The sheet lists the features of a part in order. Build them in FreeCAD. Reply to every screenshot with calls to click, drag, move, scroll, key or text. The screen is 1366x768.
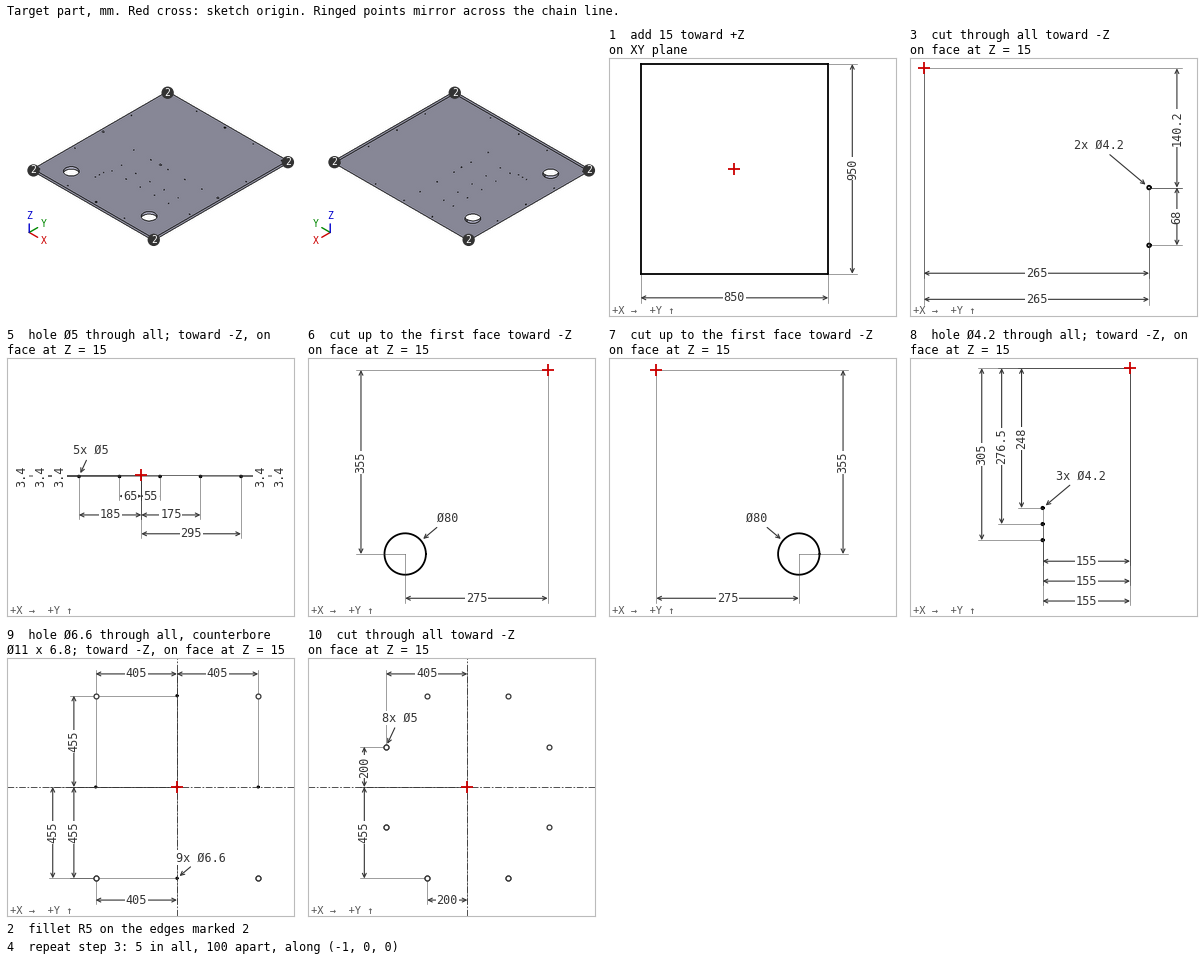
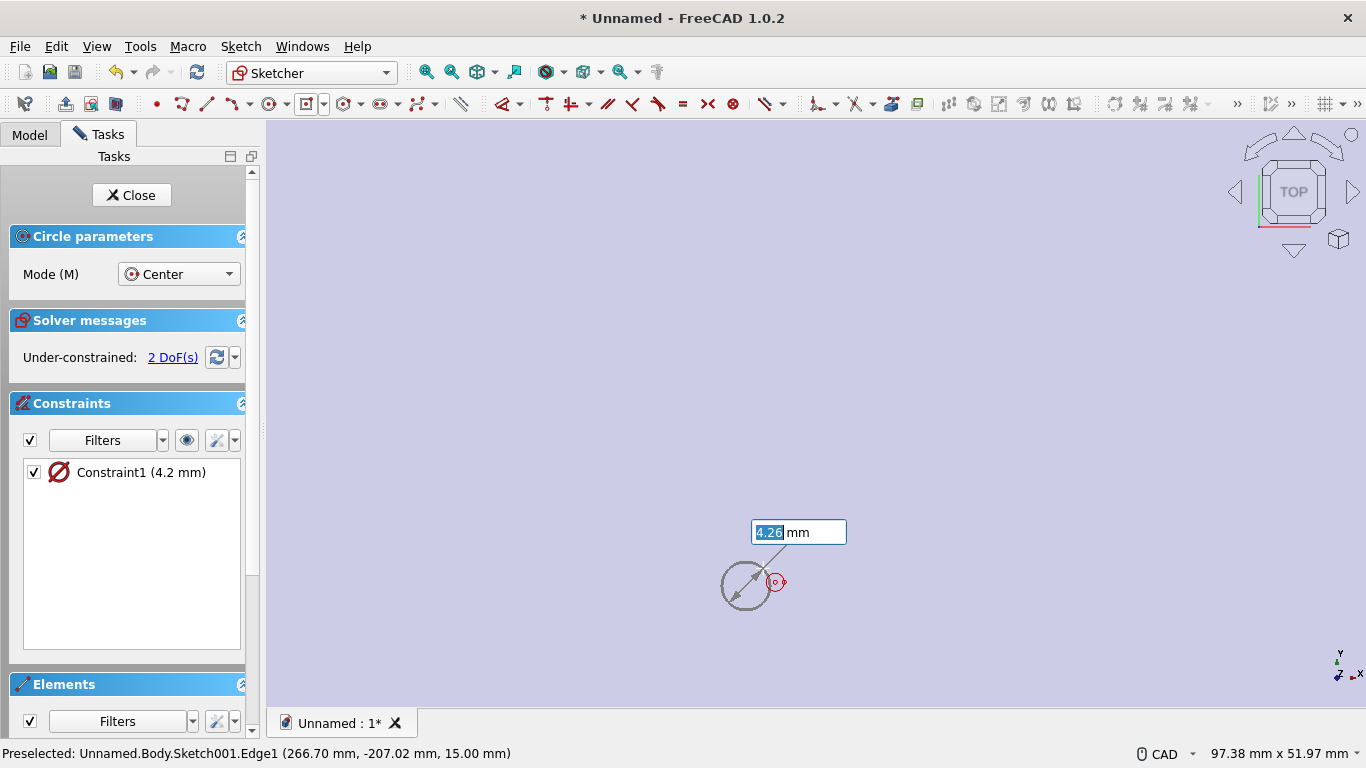
text(4.2)
key(Return)
key(Escape)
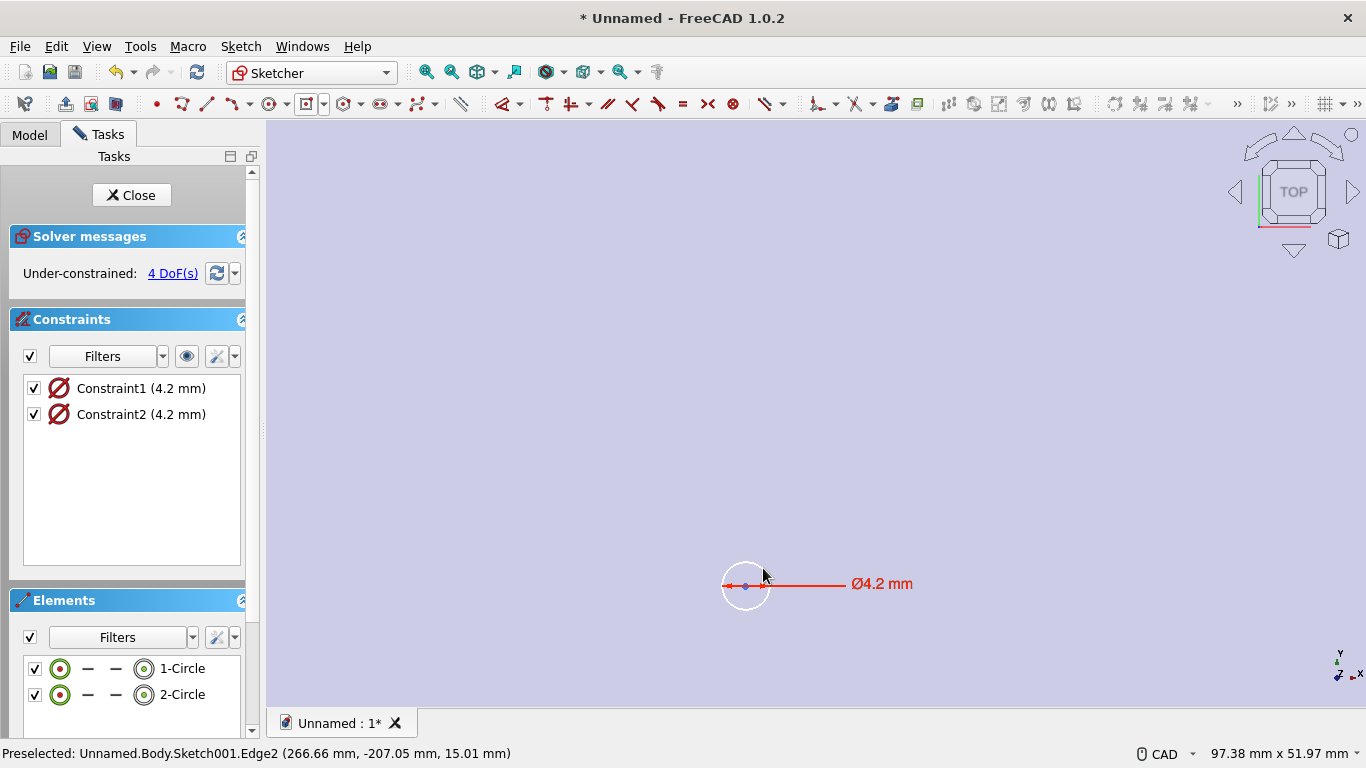
scroll(748, 587, down, 4)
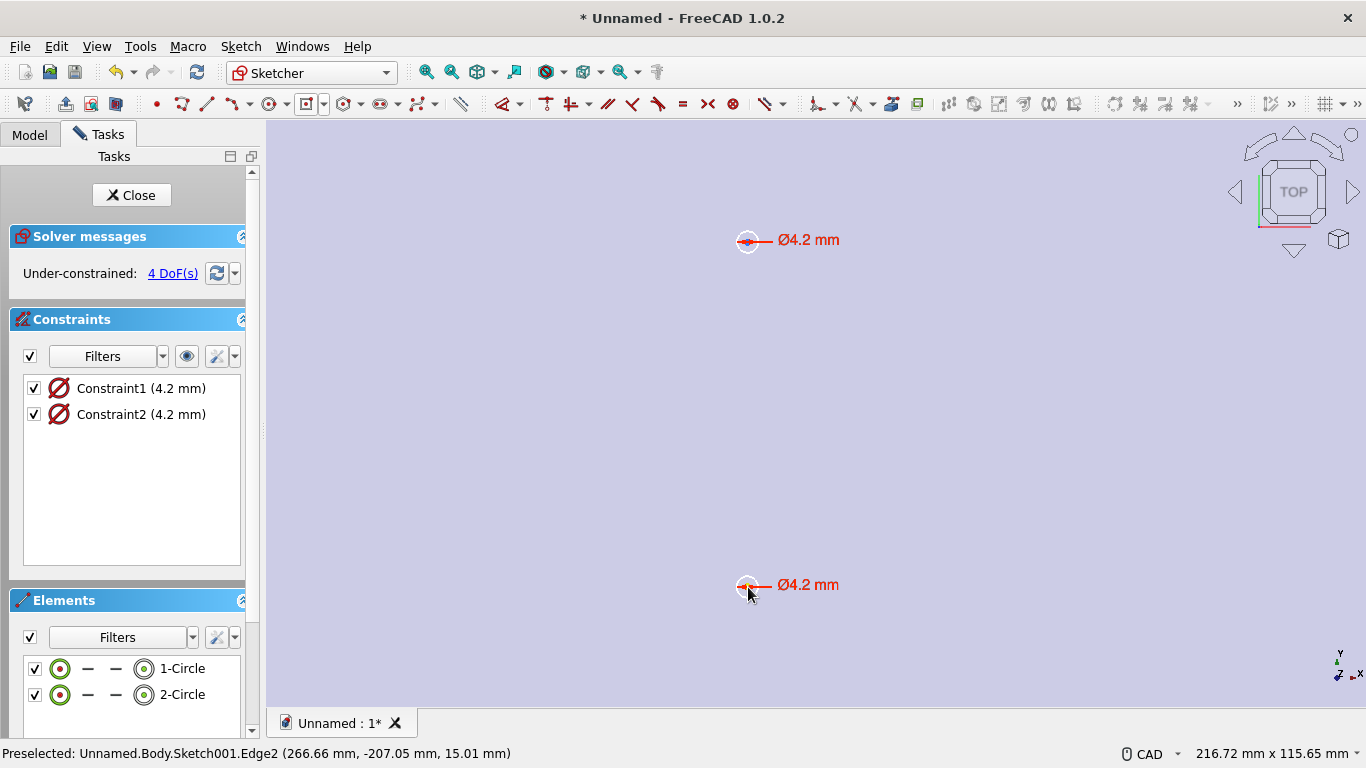
click(748, 242)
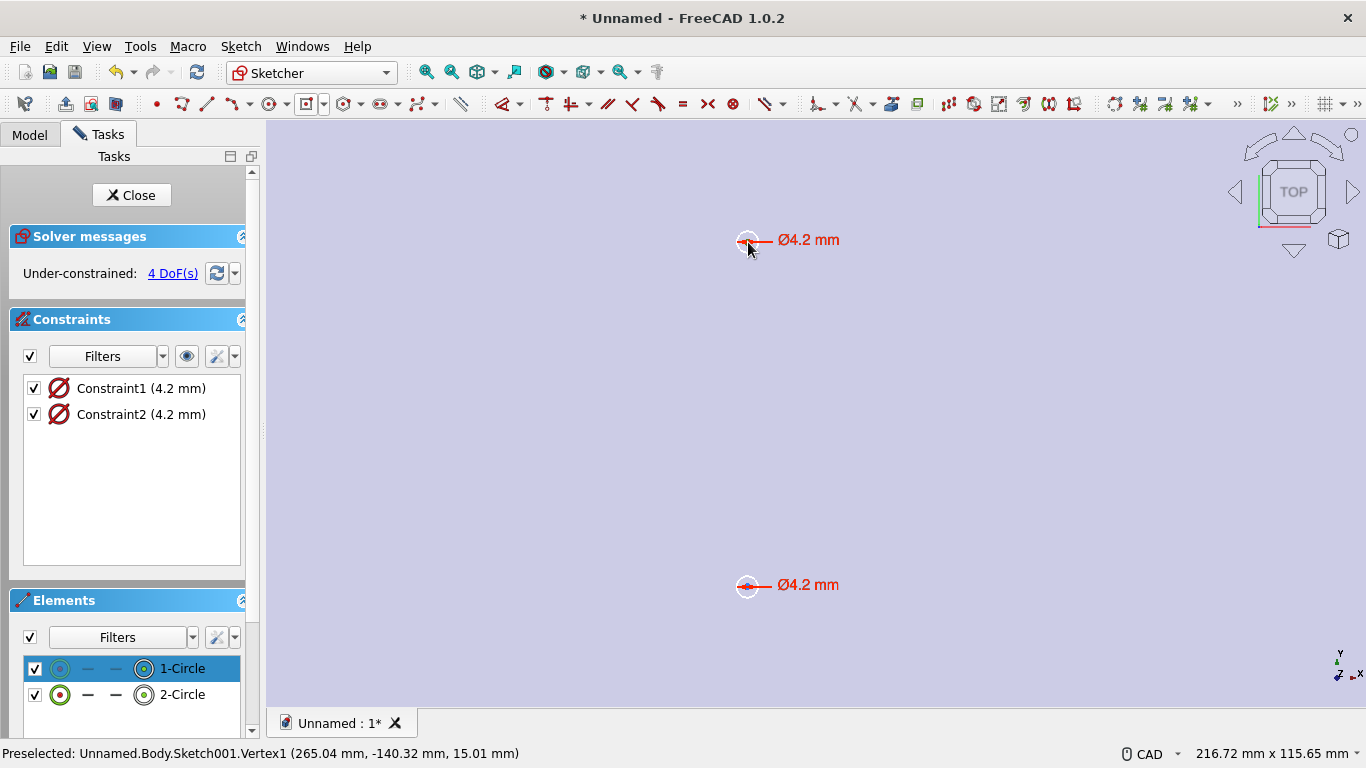
key(l)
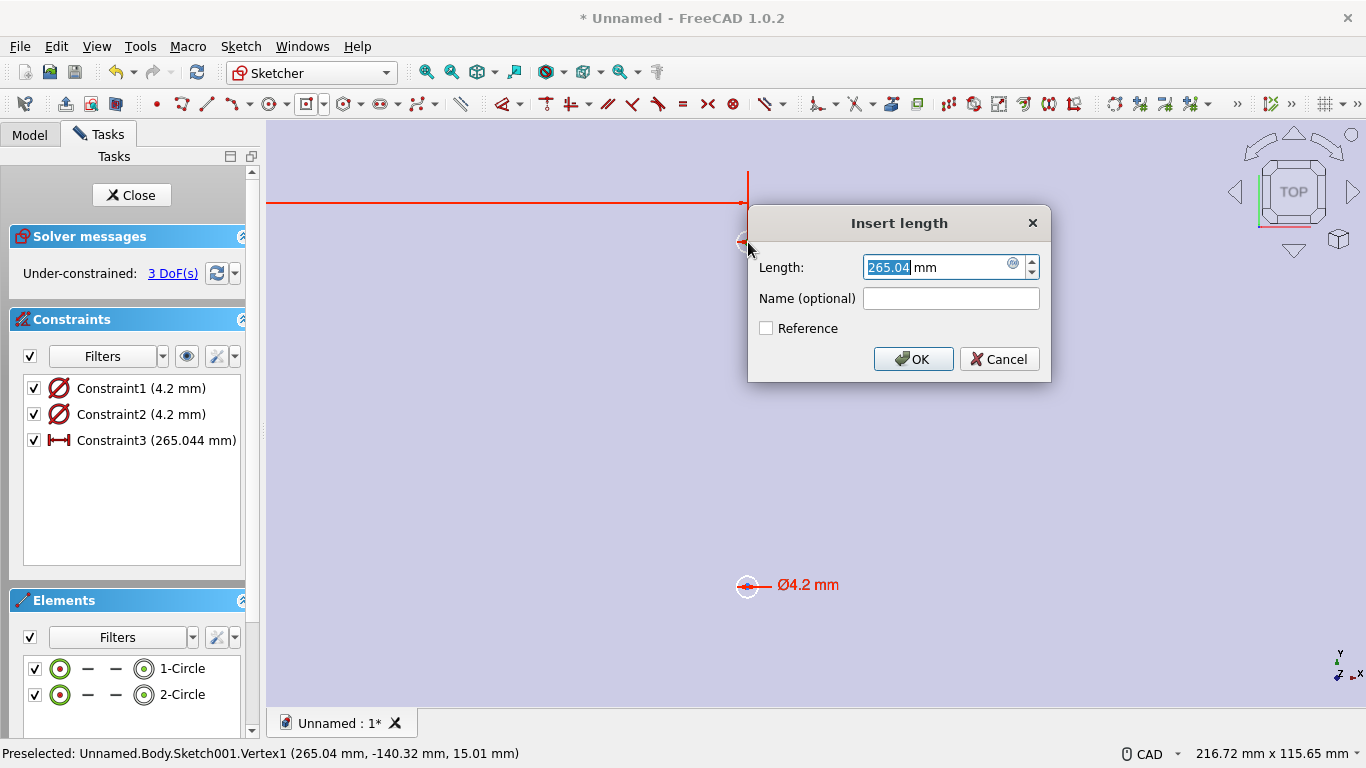
text(265)
key(Return)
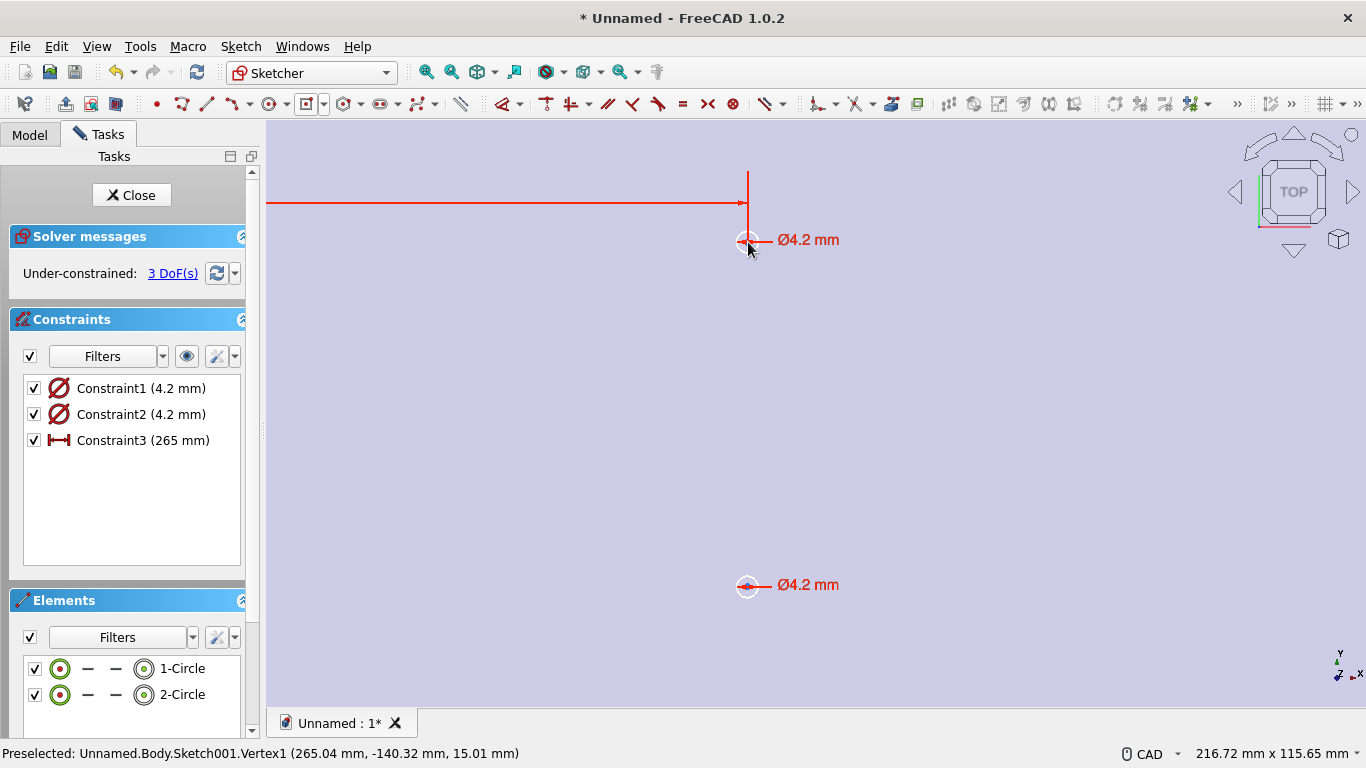
click(747, 587)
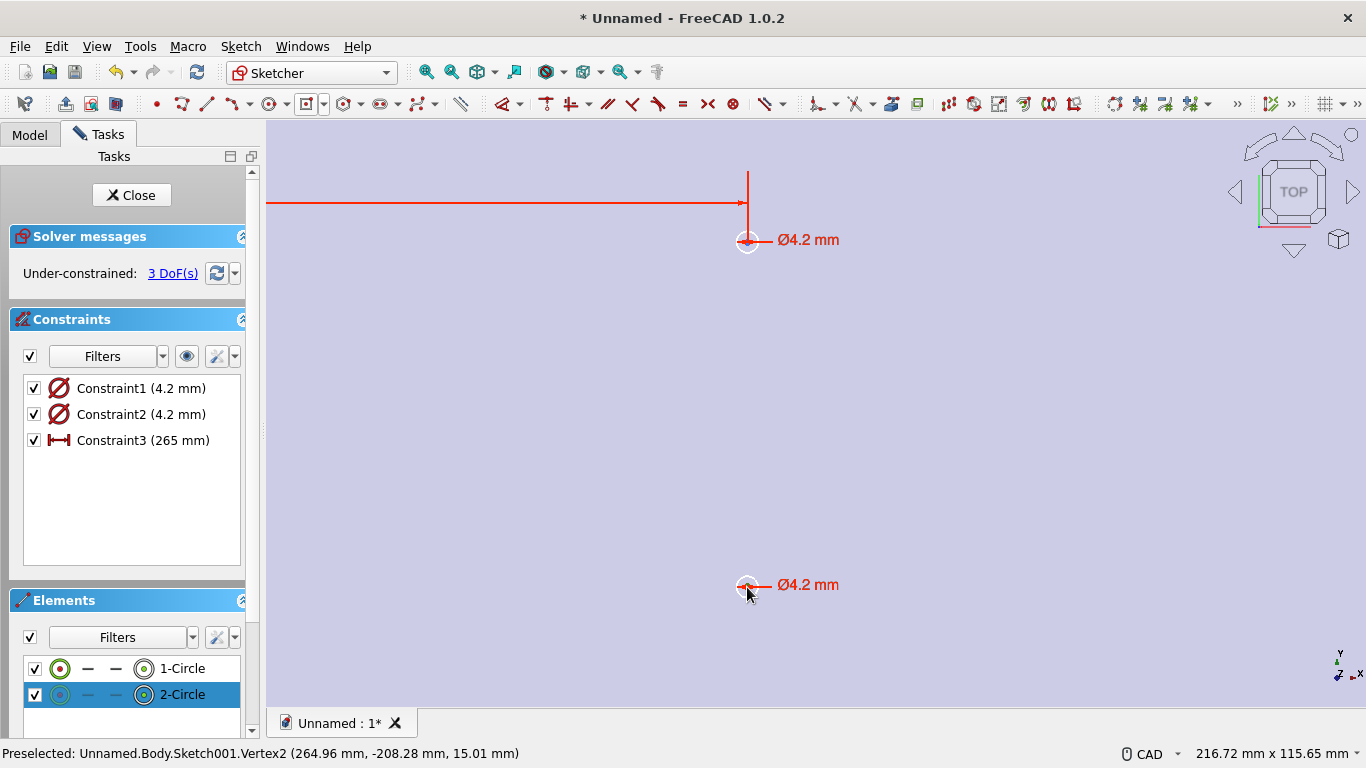
key(l)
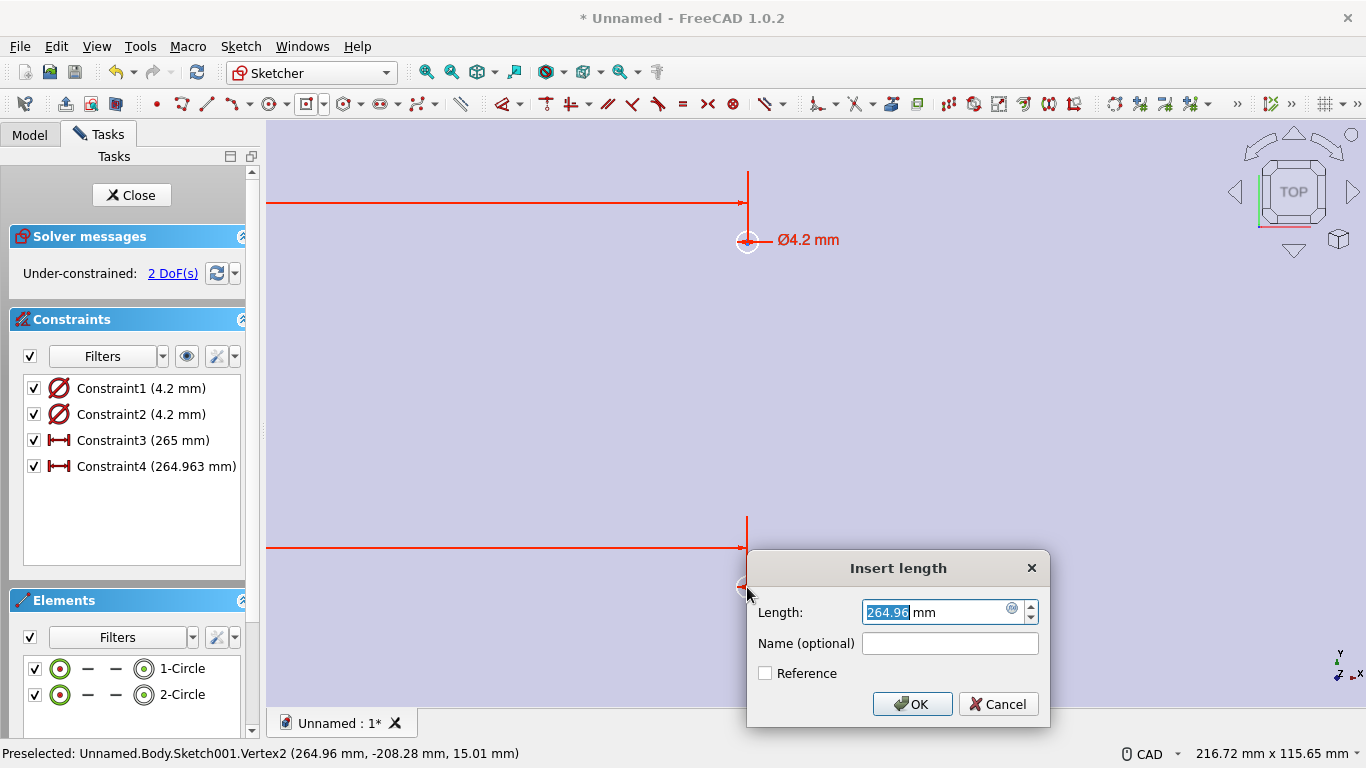
text(265)
key(Return)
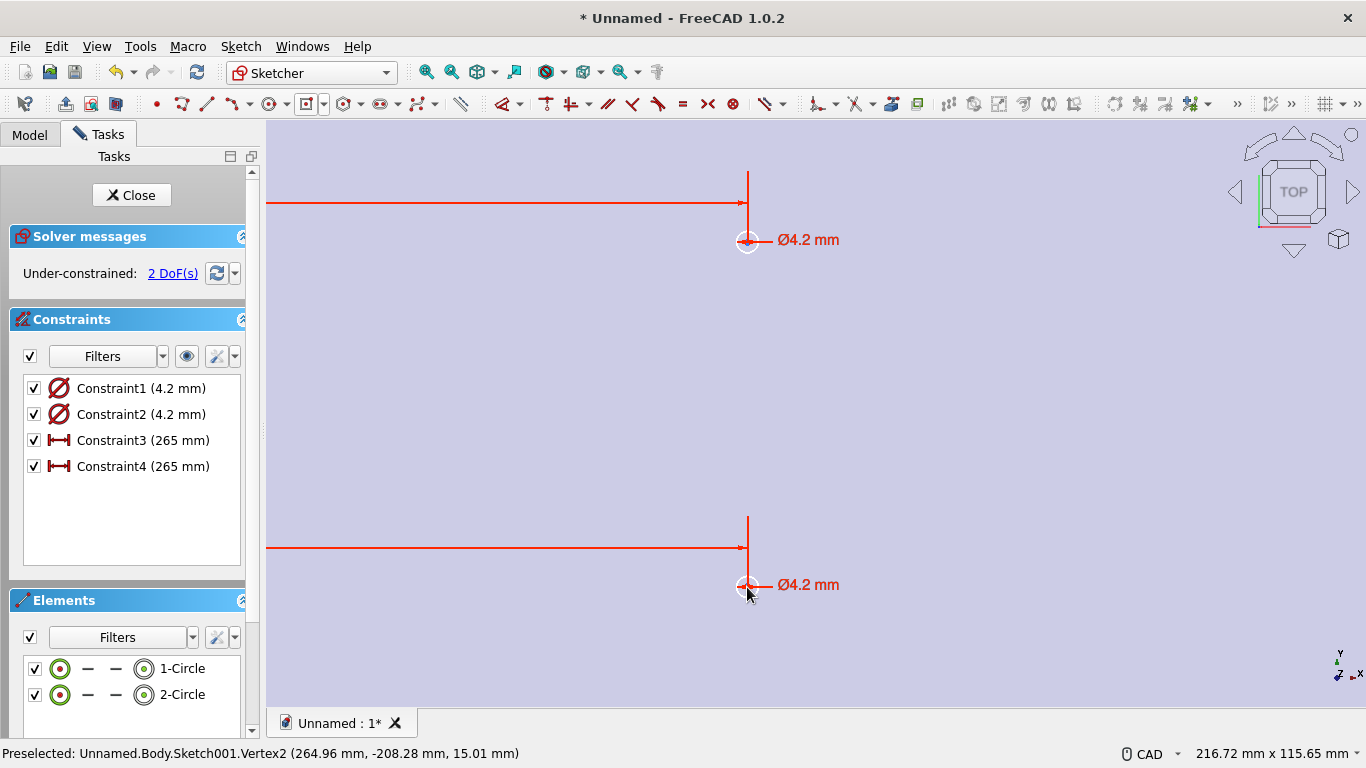
click(748, 242)